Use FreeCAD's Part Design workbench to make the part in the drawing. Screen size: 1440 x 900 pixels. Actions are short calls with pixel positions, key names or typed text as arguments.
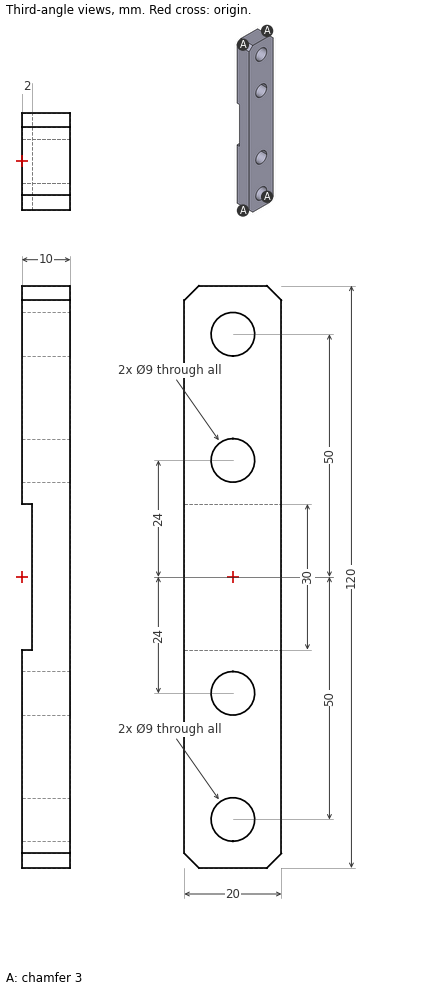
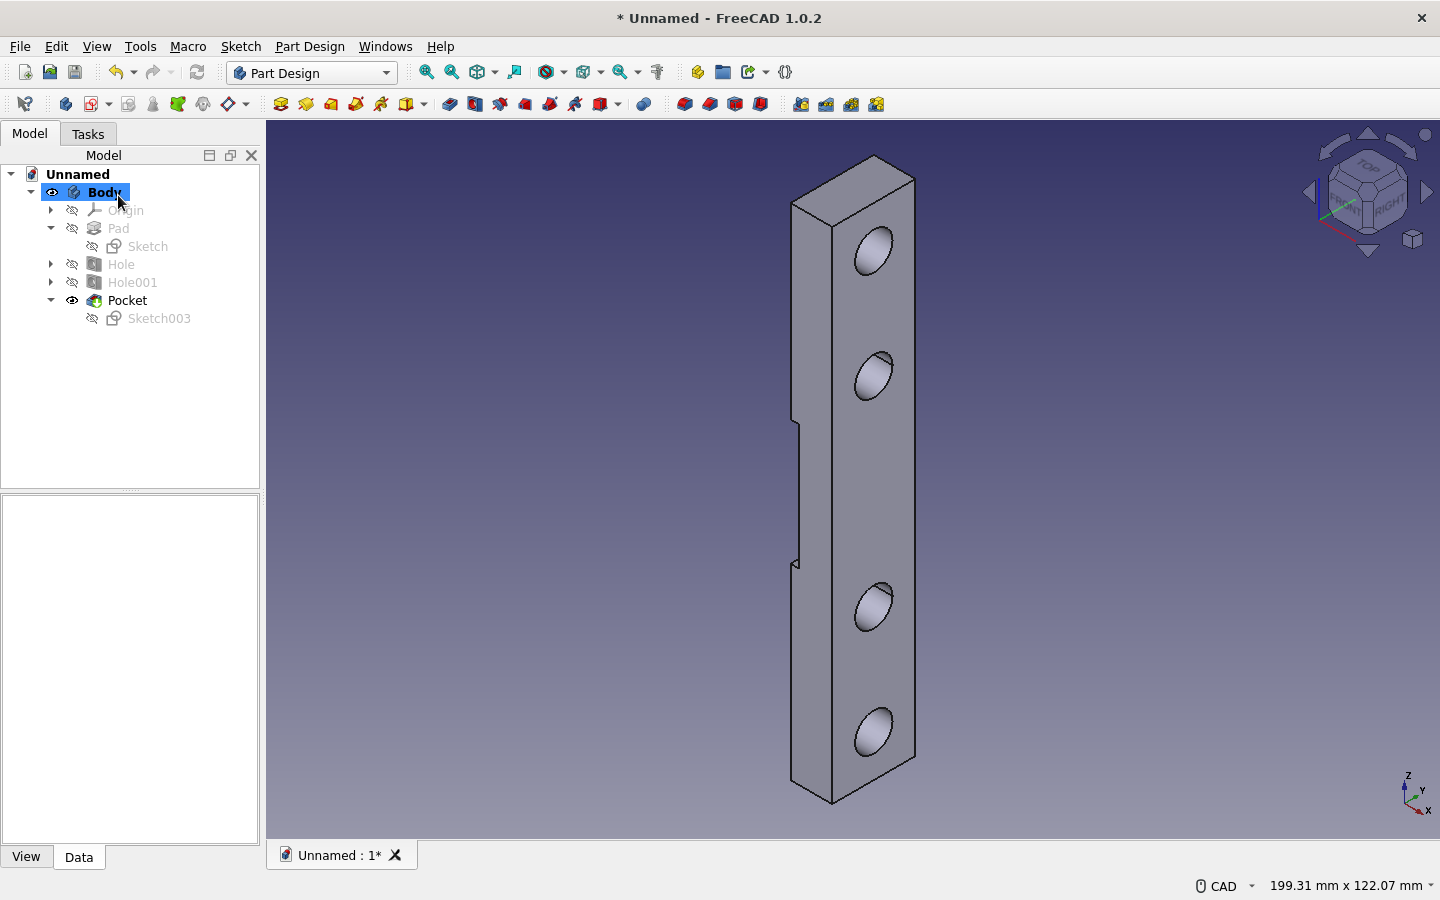
click(811, 214)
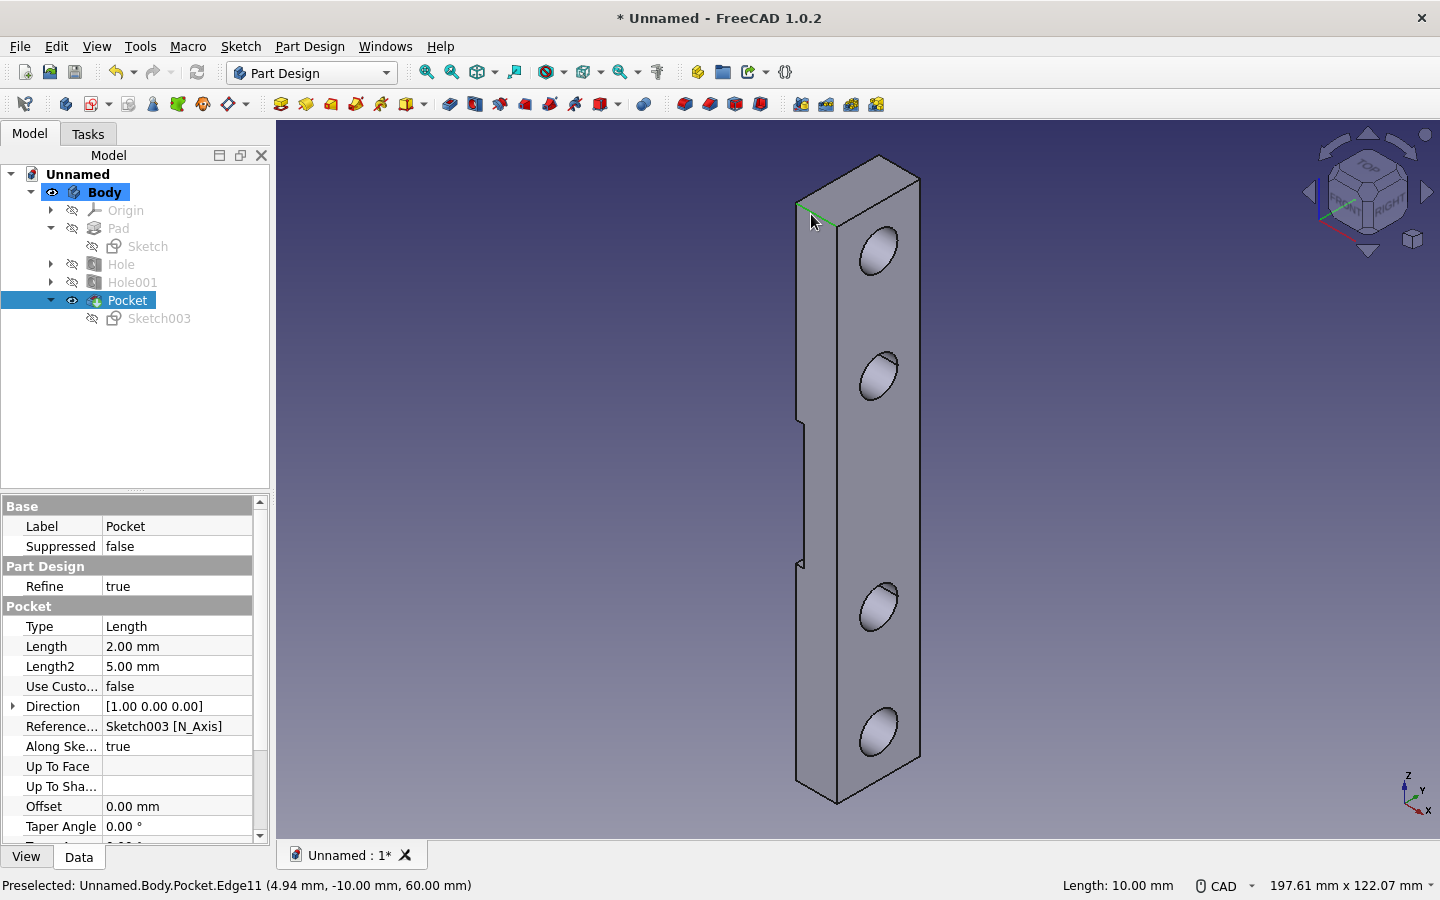
key(2)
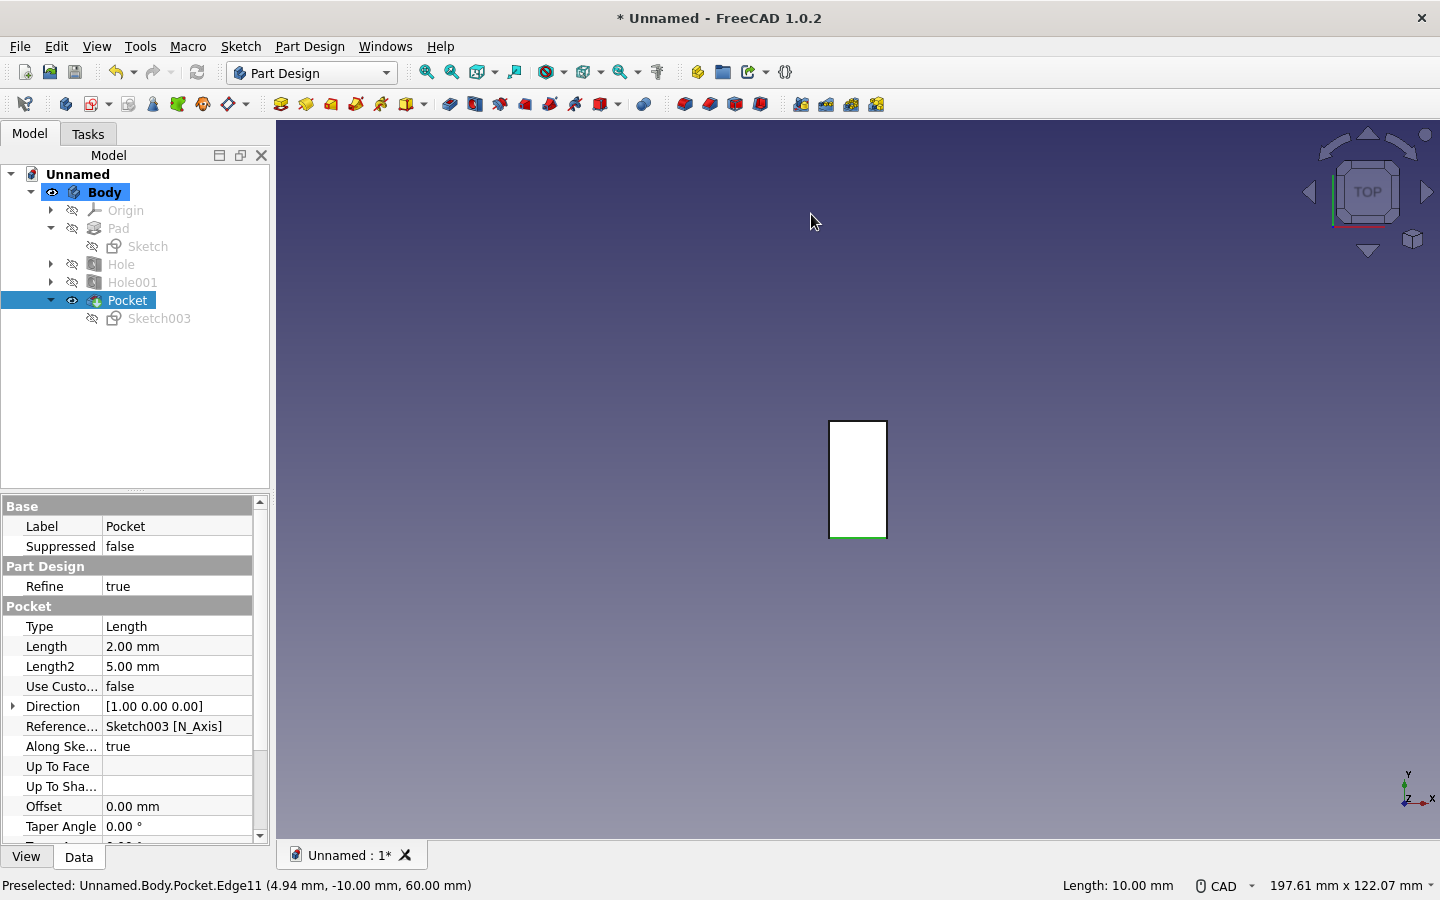
key(v)
key(f)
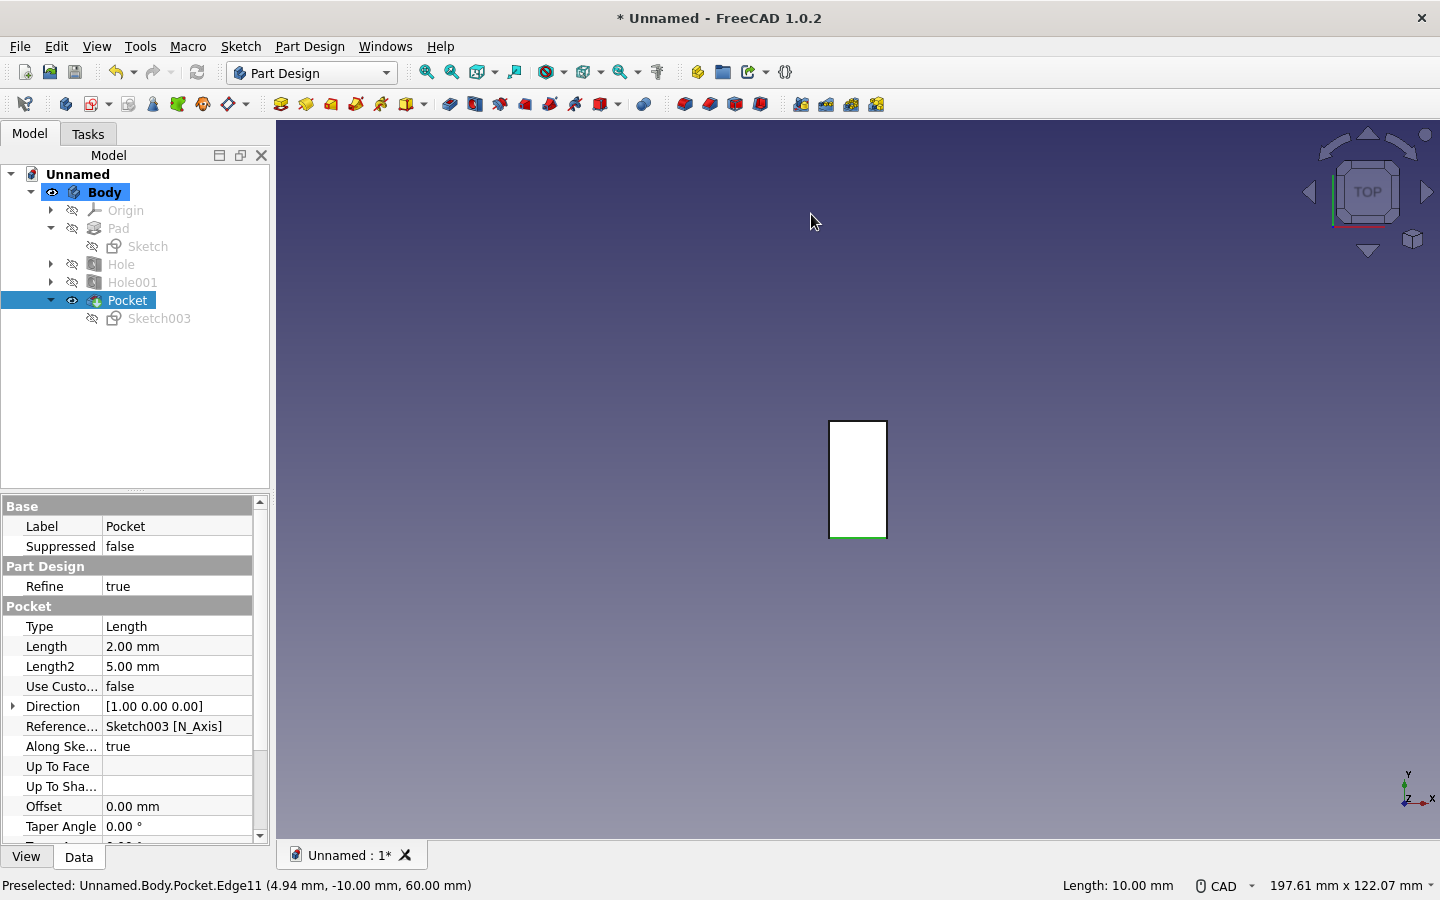
click(858, 420, ctrl)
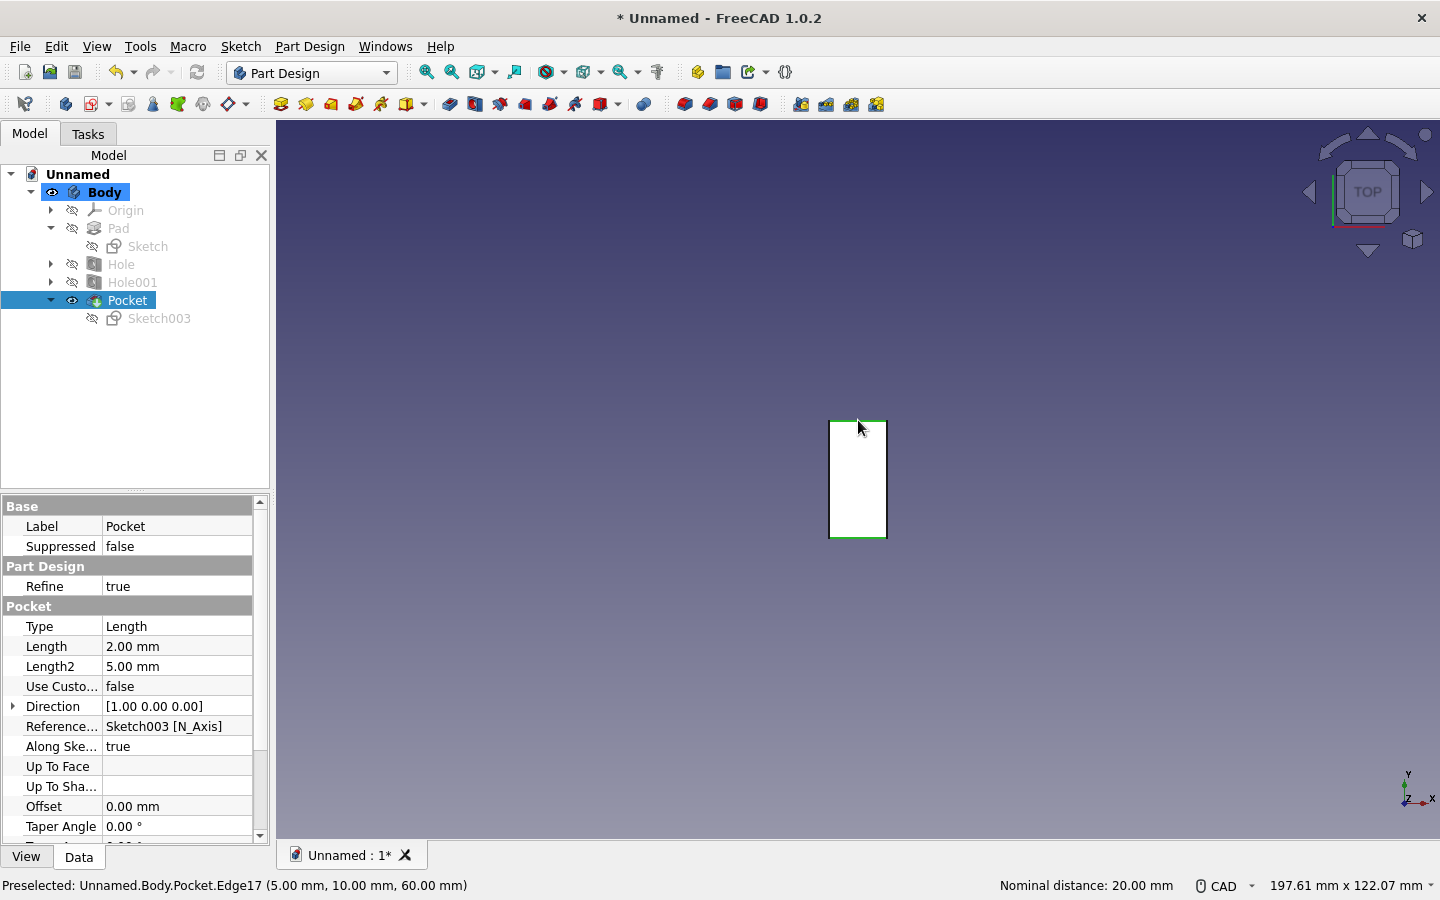
key(1)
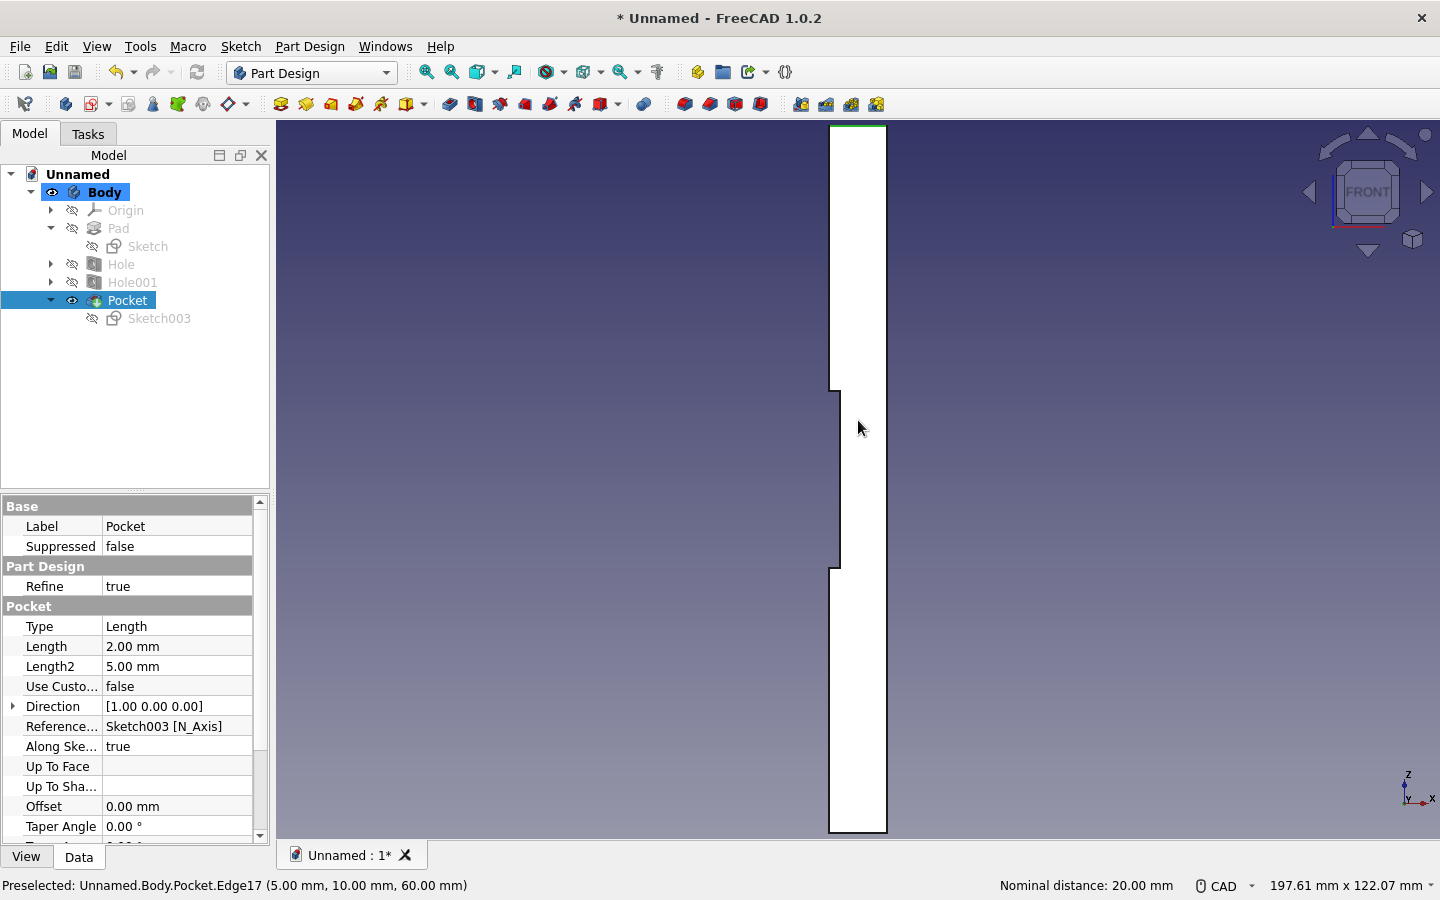
key(3)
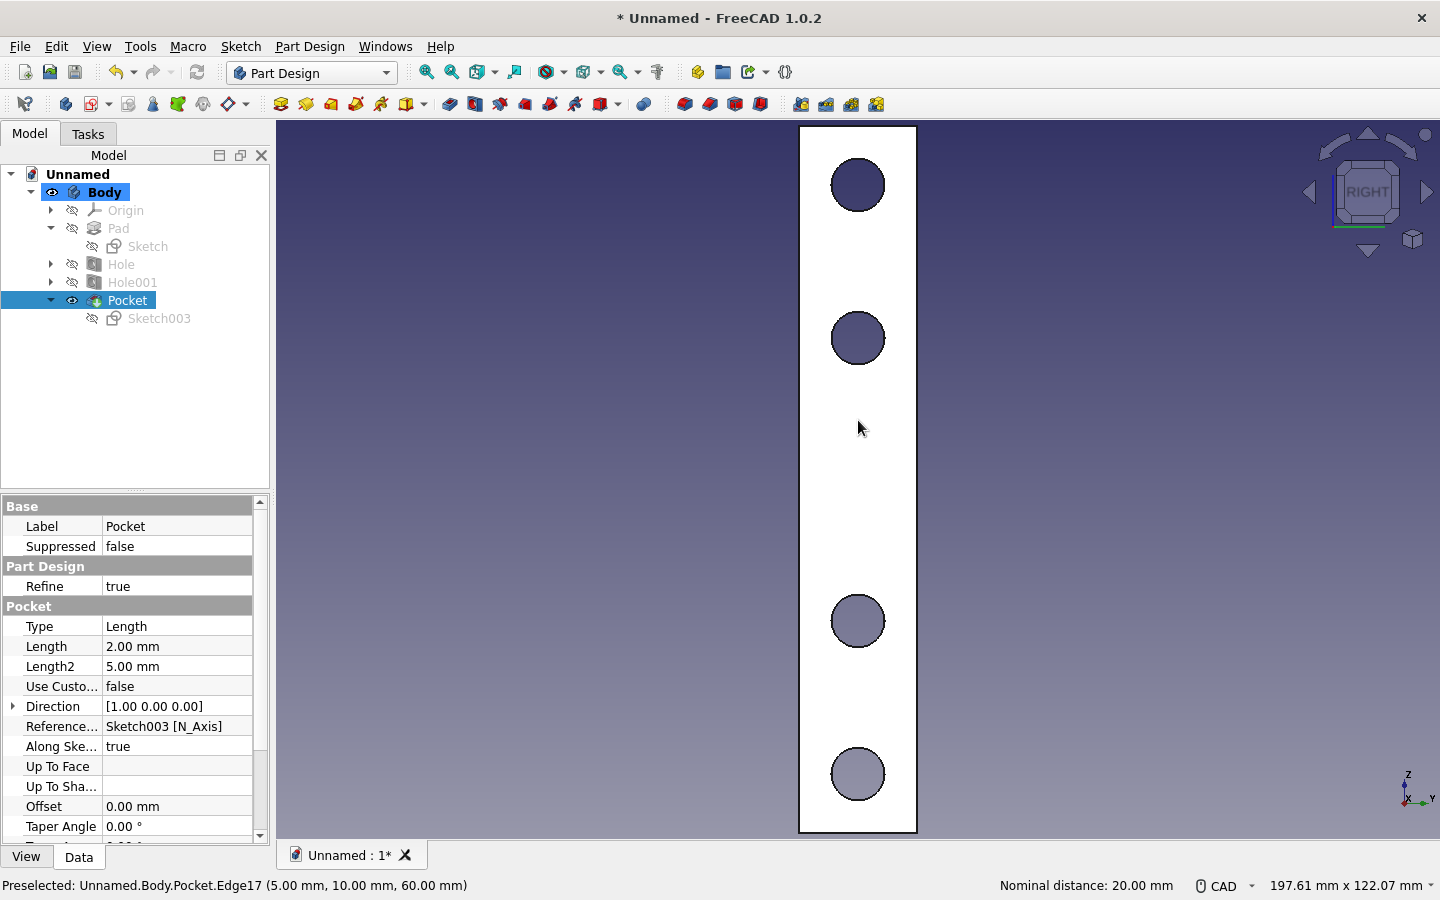
key(5)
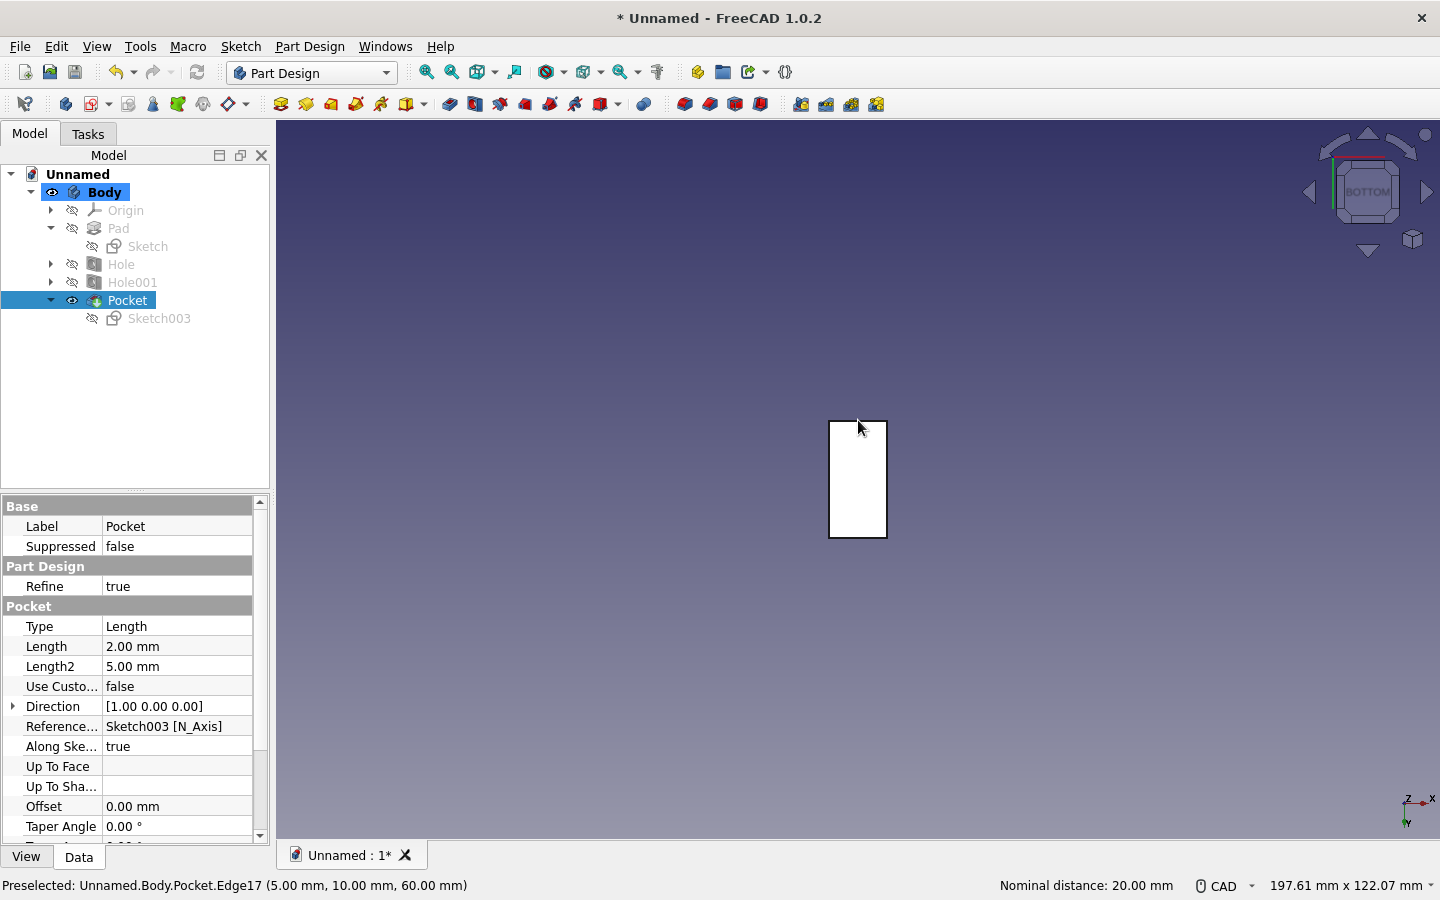
key(v)
key(f)